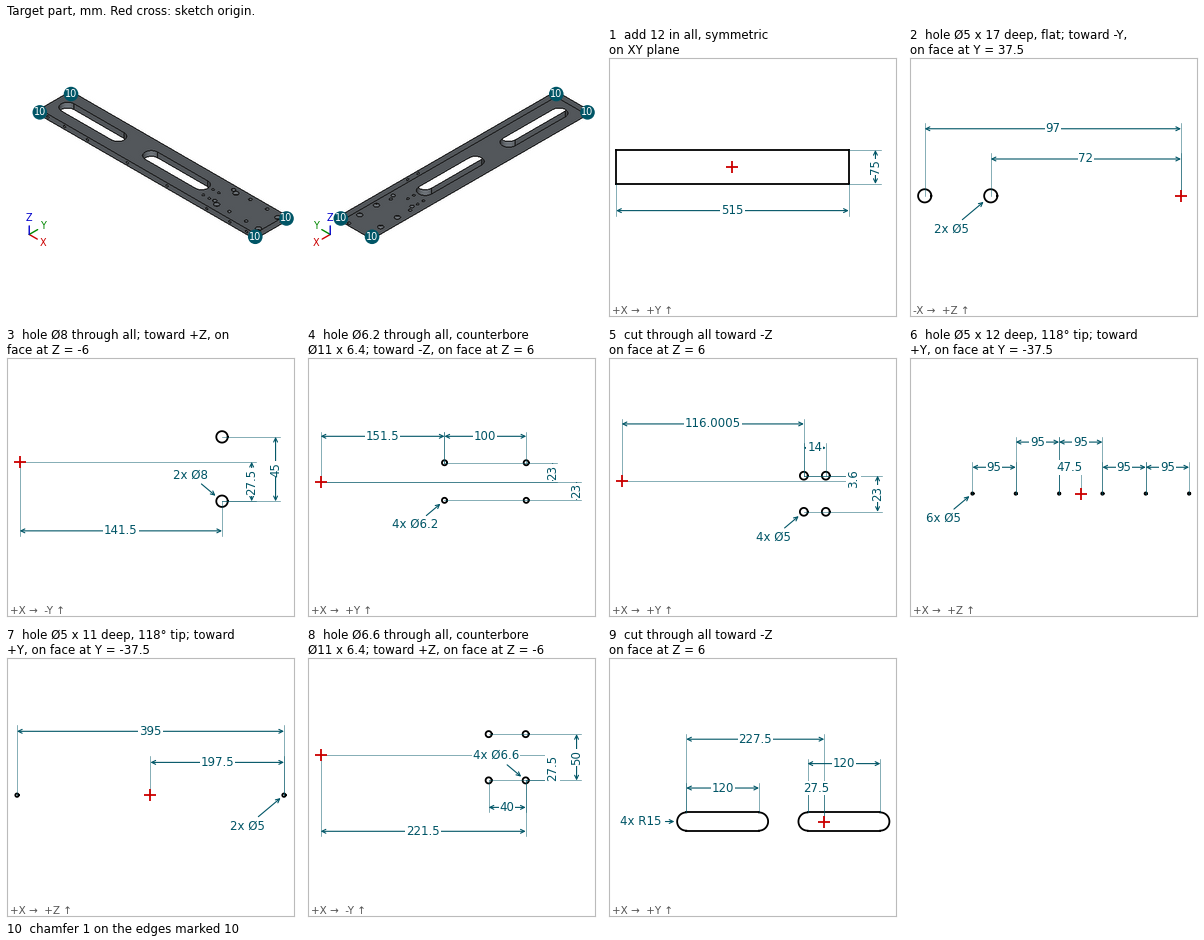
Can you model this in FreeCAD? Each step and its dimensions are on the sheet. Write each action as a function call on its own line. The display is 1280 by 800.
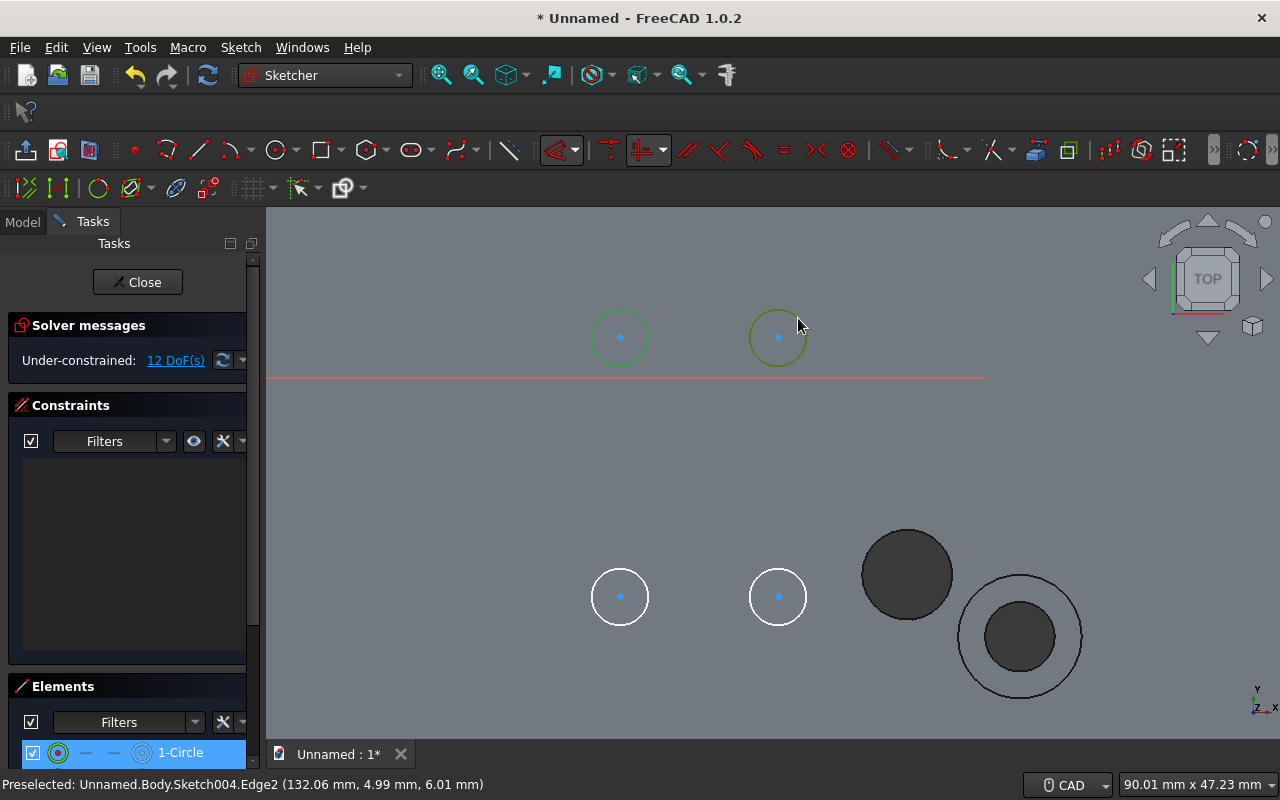
click(640, 577)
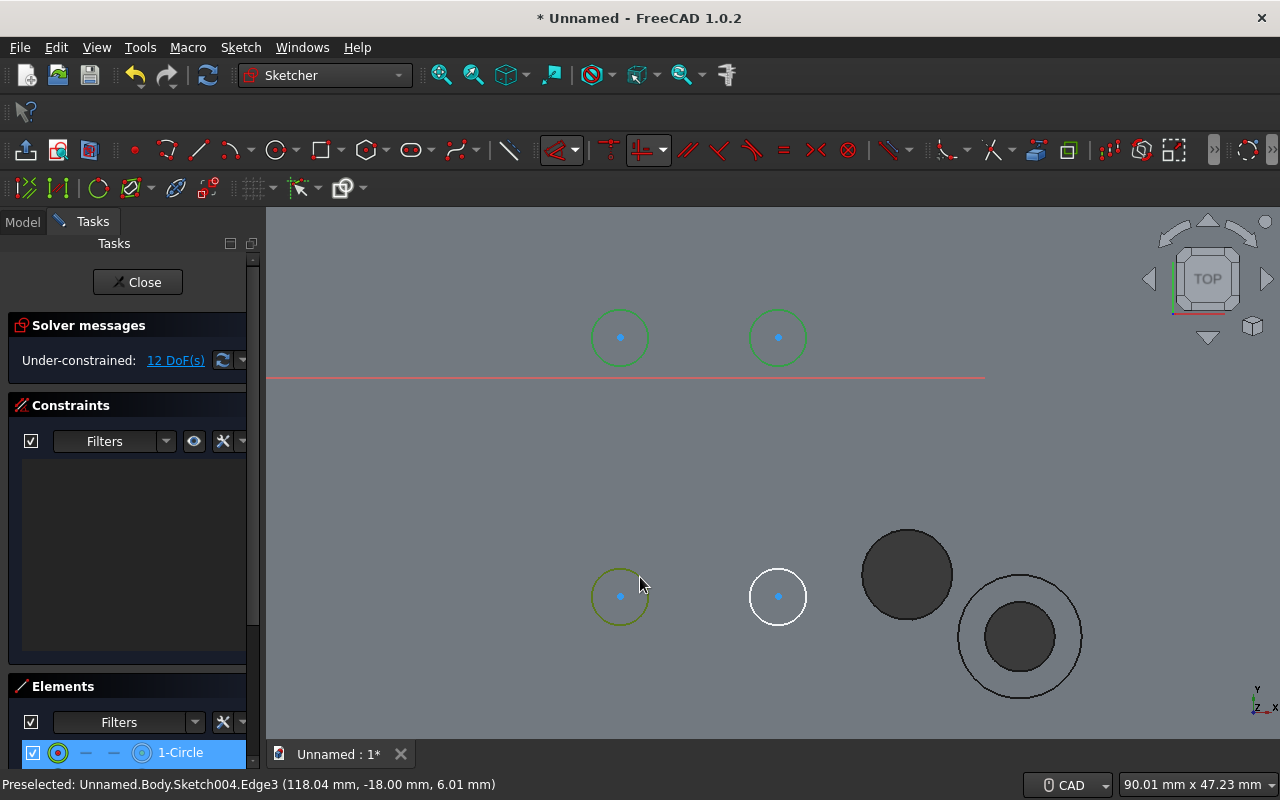
click(798, 577)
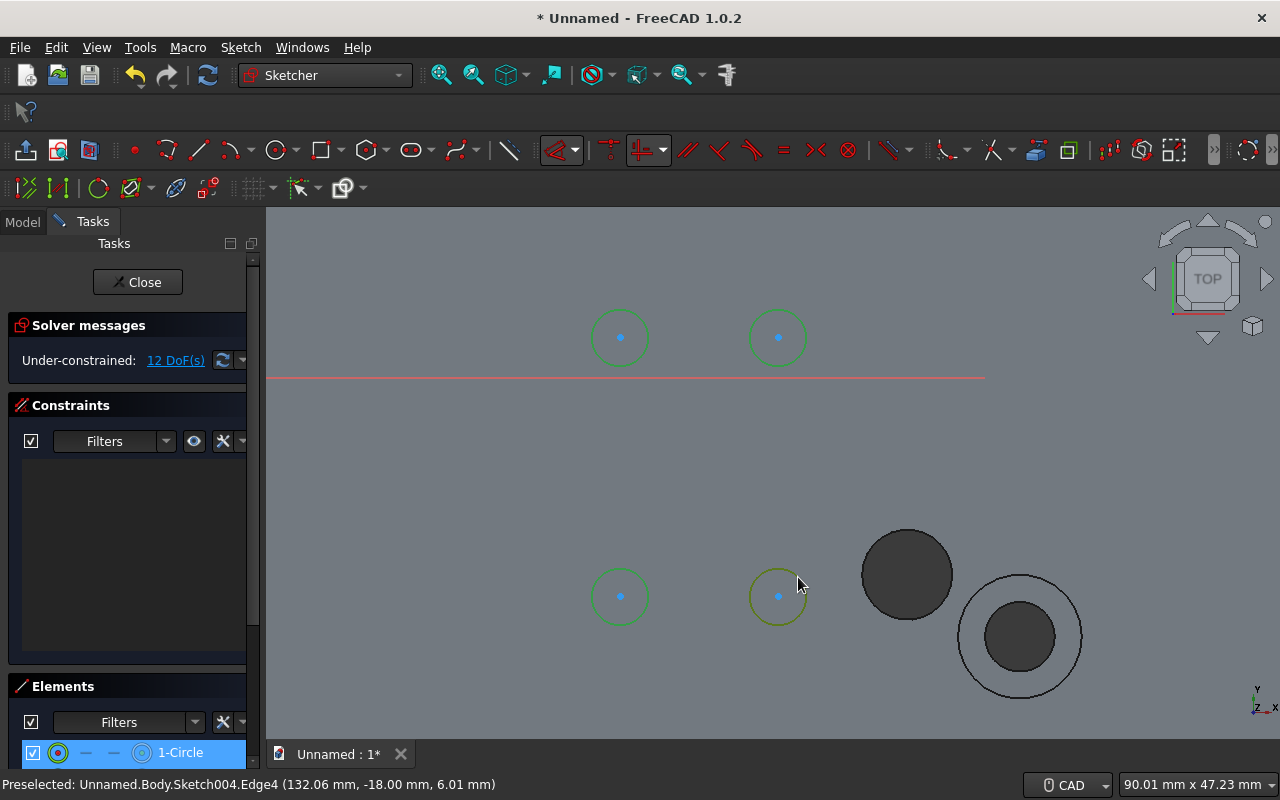
key(e)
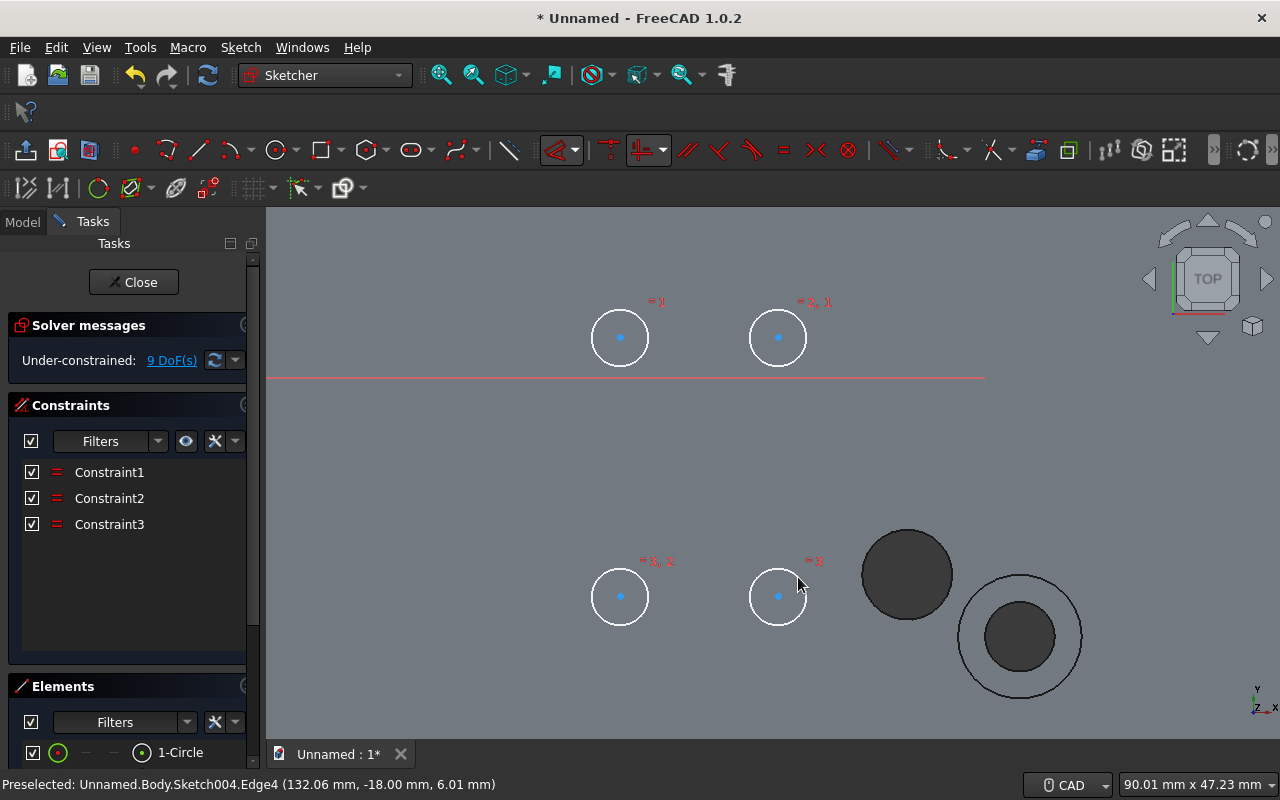
click(620, 338)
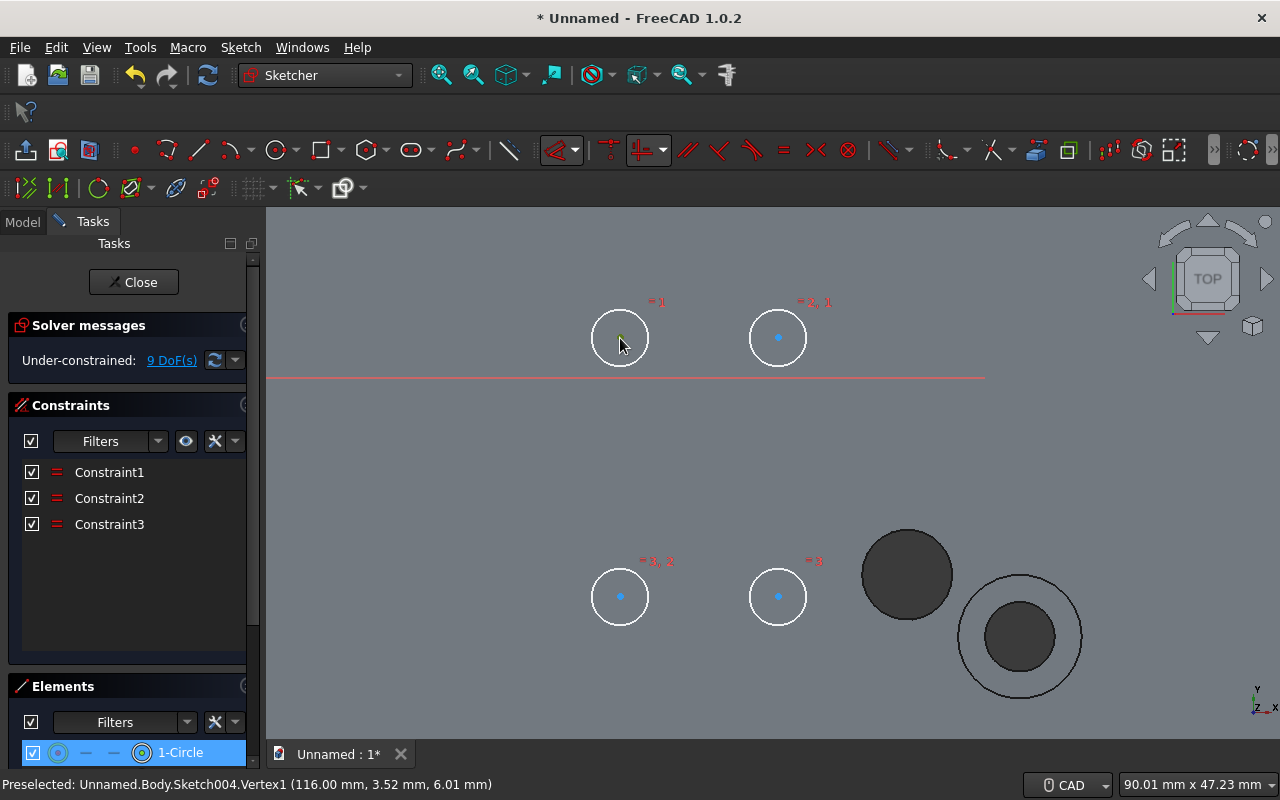
click(778, 338)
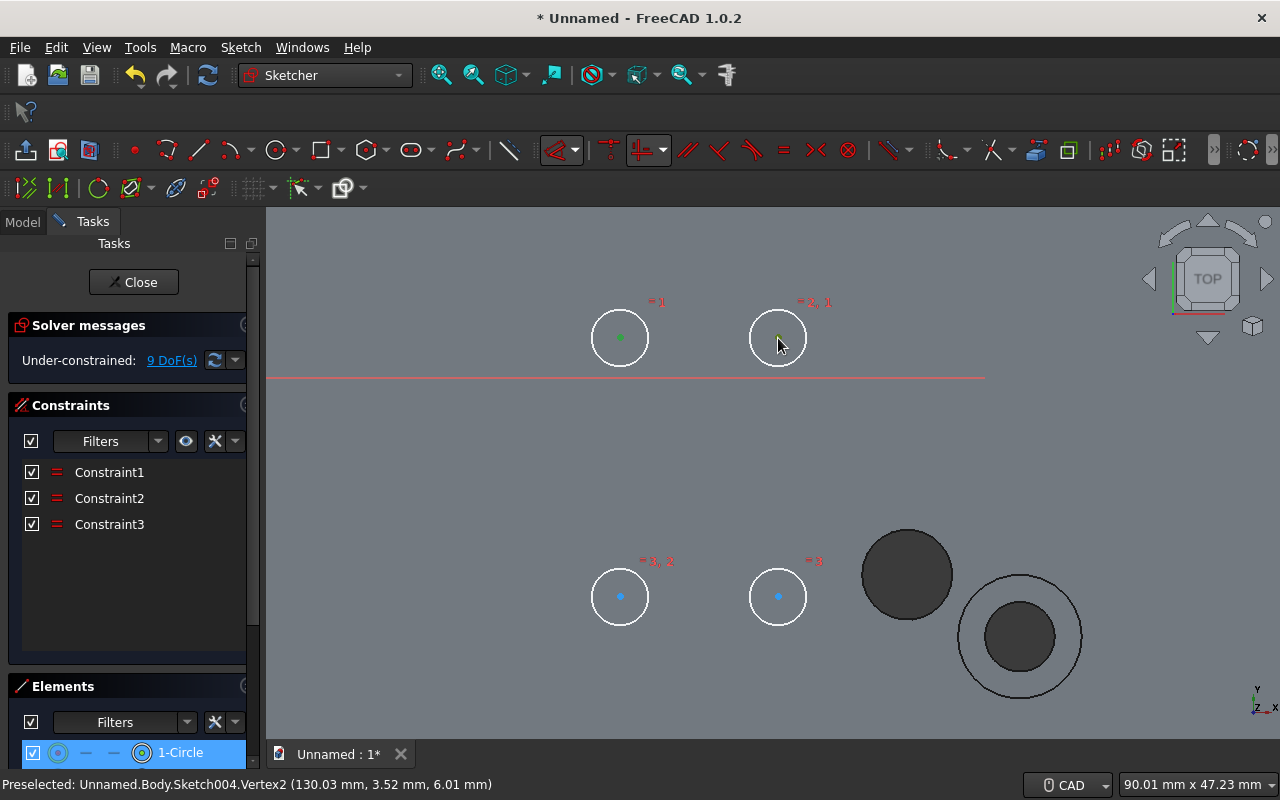
key(h)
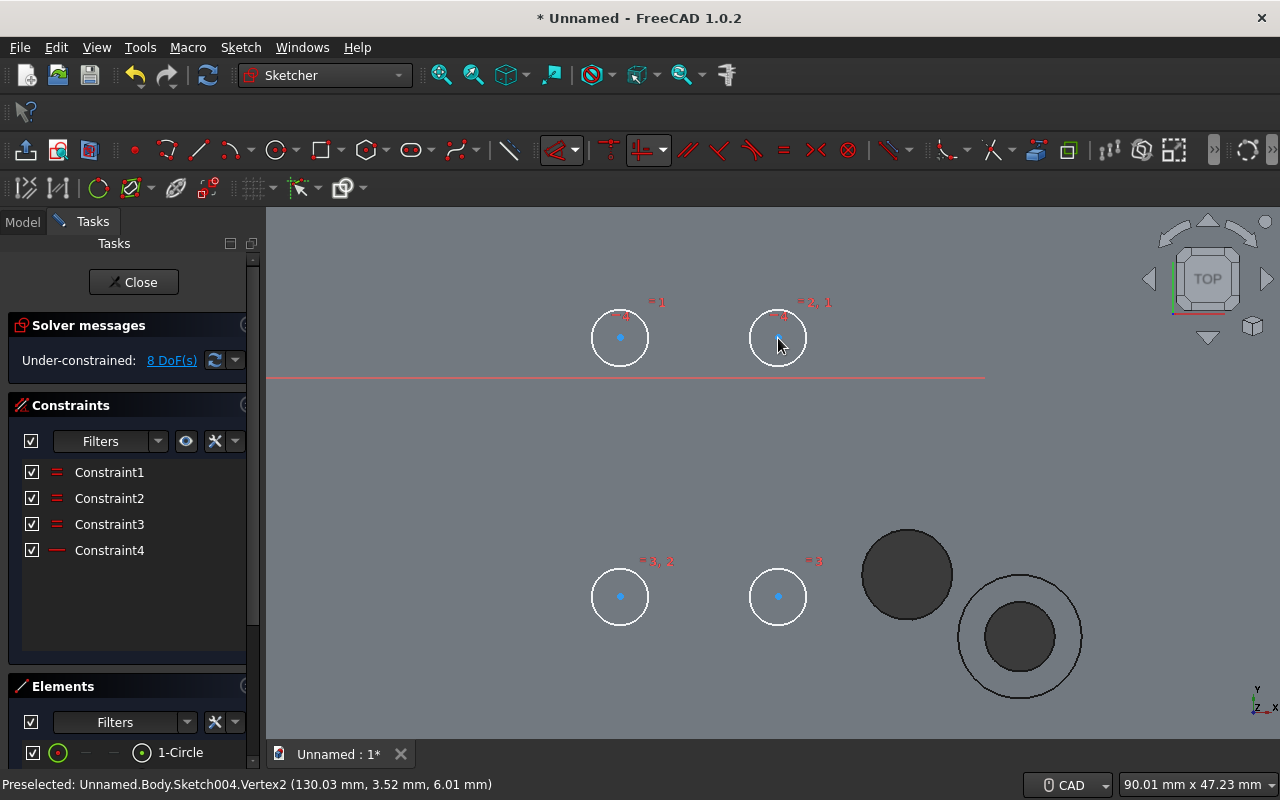
click(620, 338)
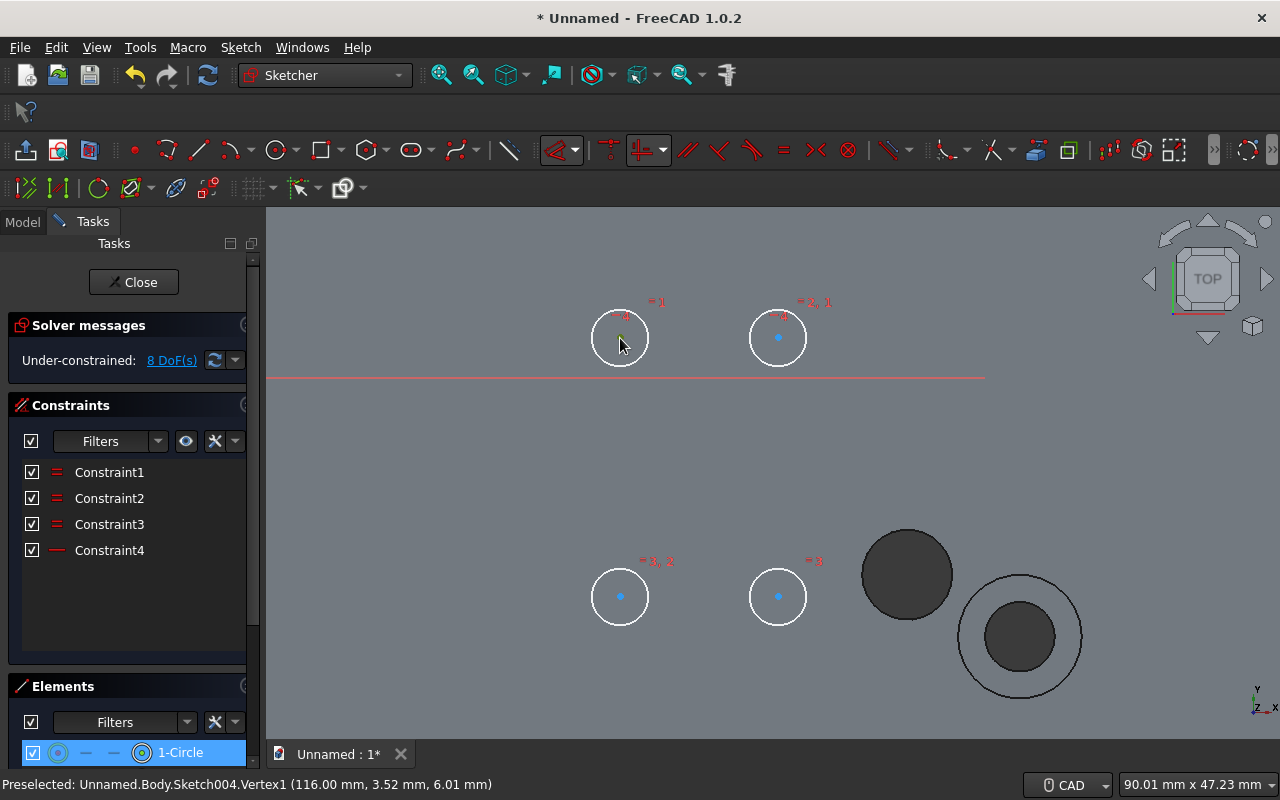
click(620, 597)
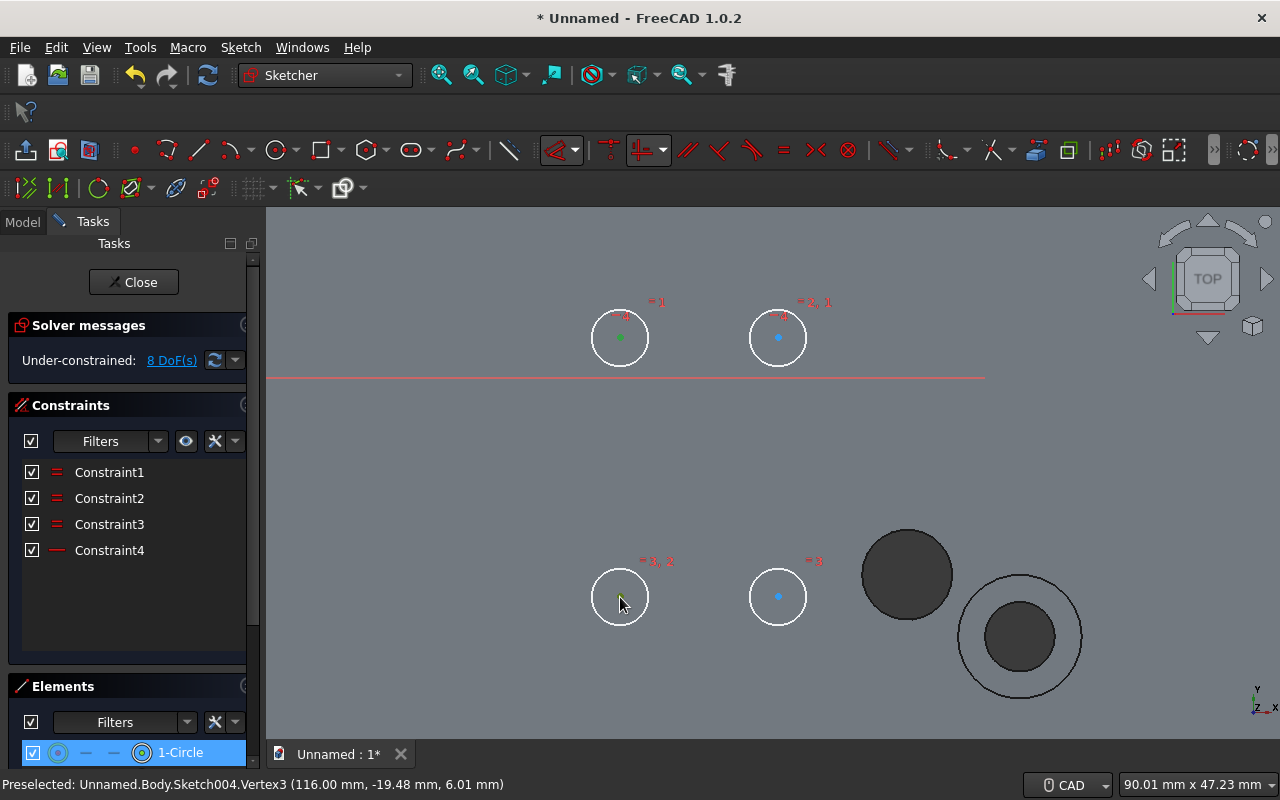
key(v)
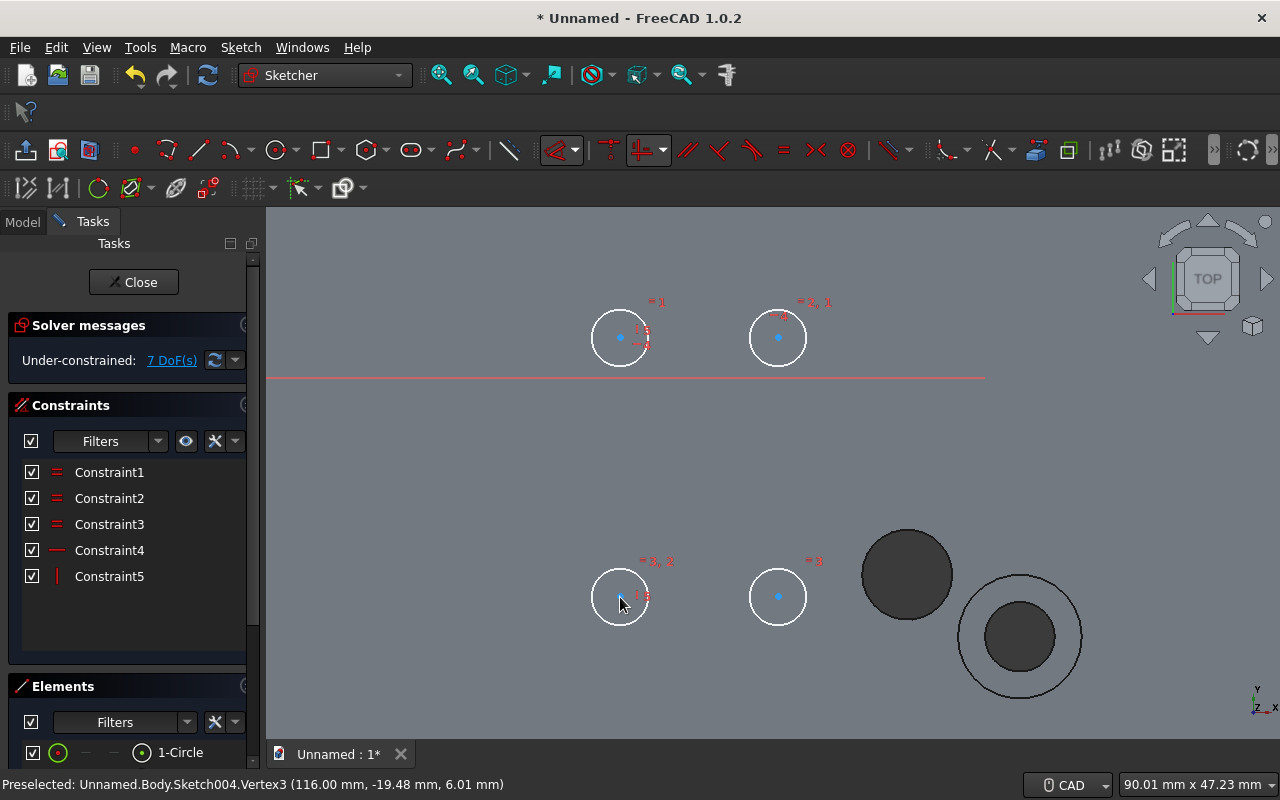
click(778, 338)